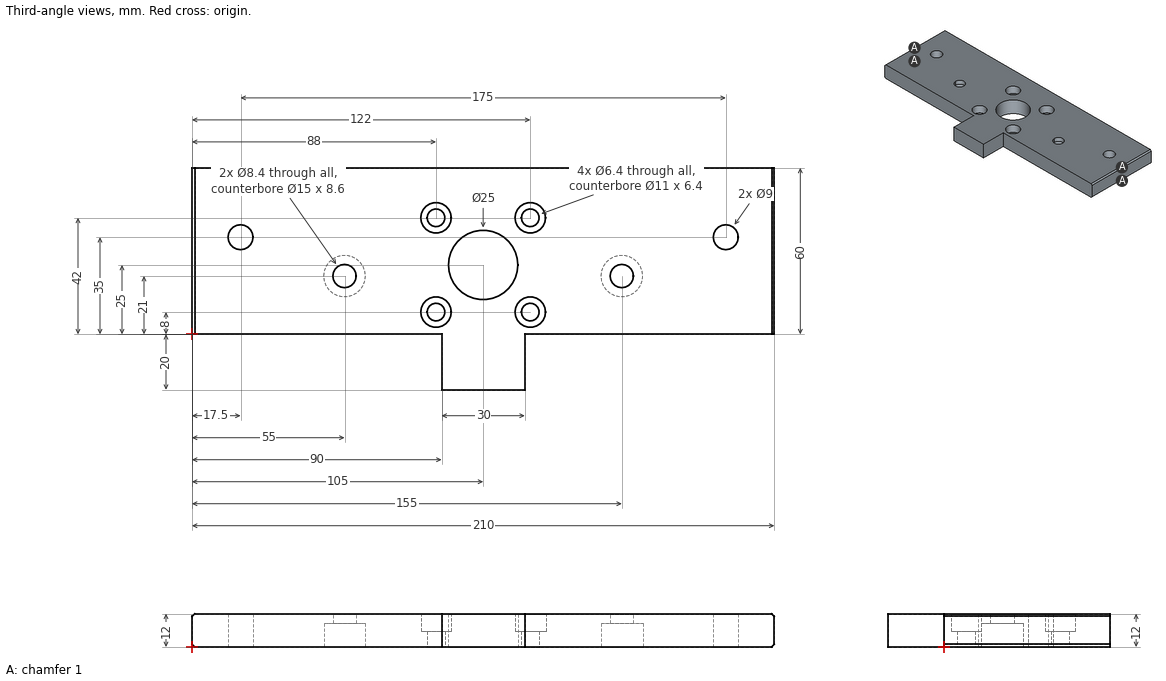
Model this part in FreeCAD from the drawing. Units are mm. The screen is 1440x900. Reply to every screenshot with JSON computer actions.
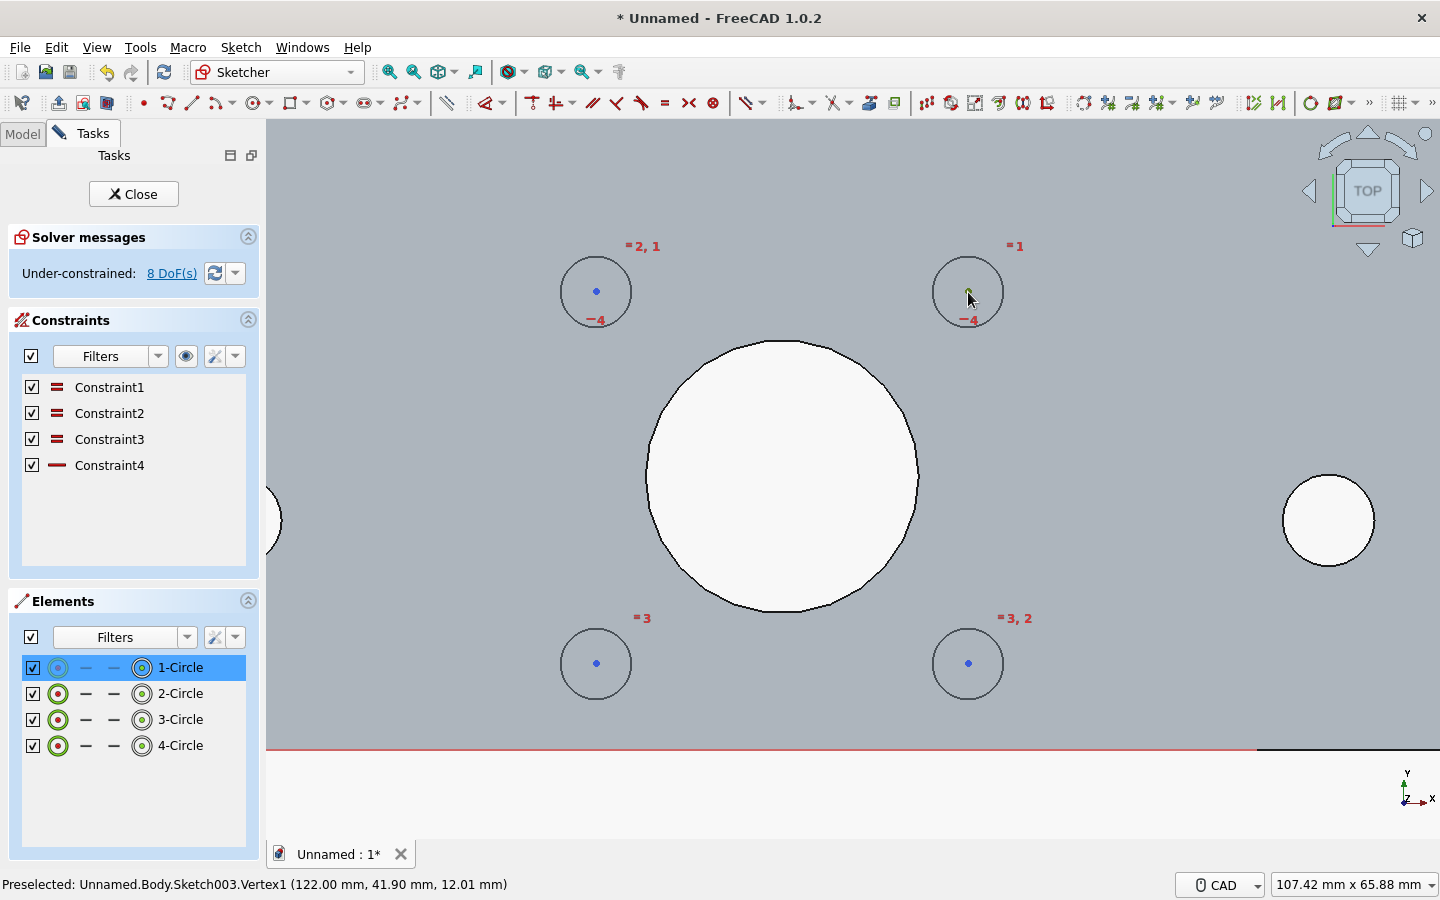
{"action": "left_click", "coordinate": [968, 664]}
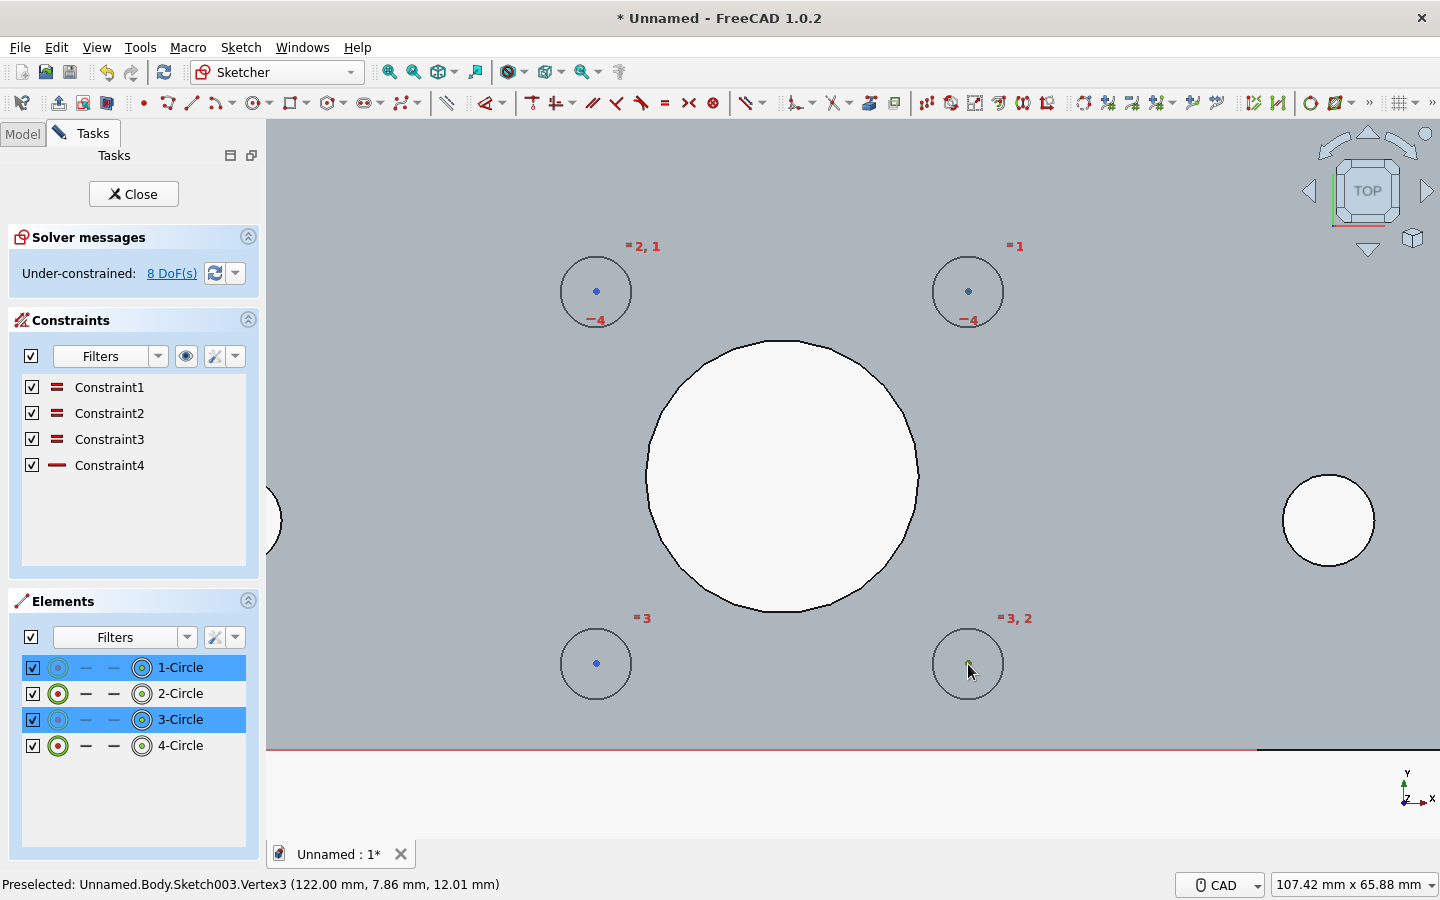
{"action": "key", "text": "v"}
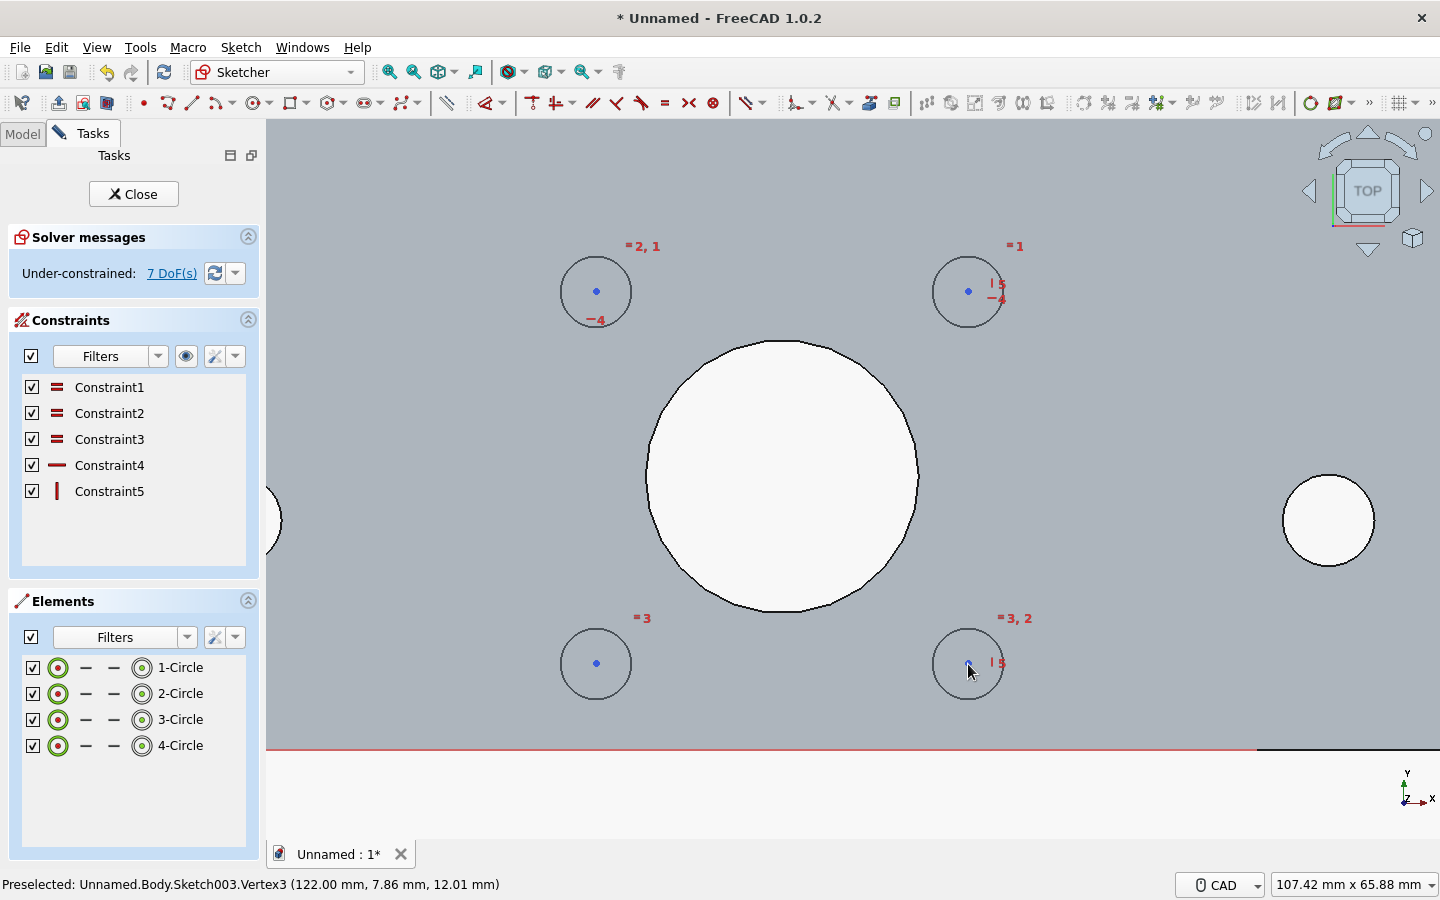
{"action": "left_click", "coordinate": [596, 292]}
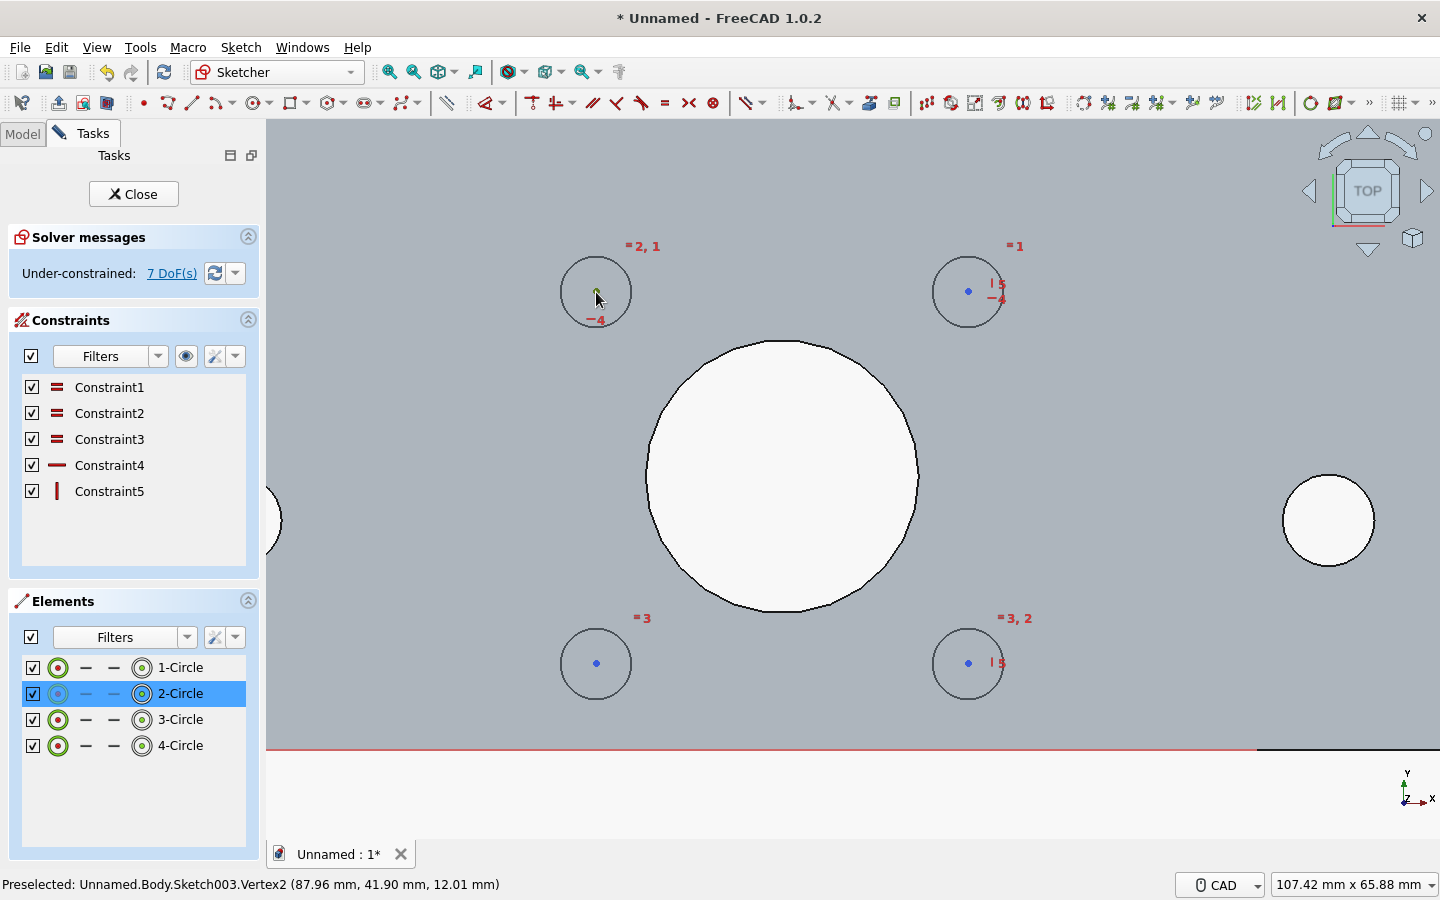
{"action": "left_click", "coordinate": [596, 664]}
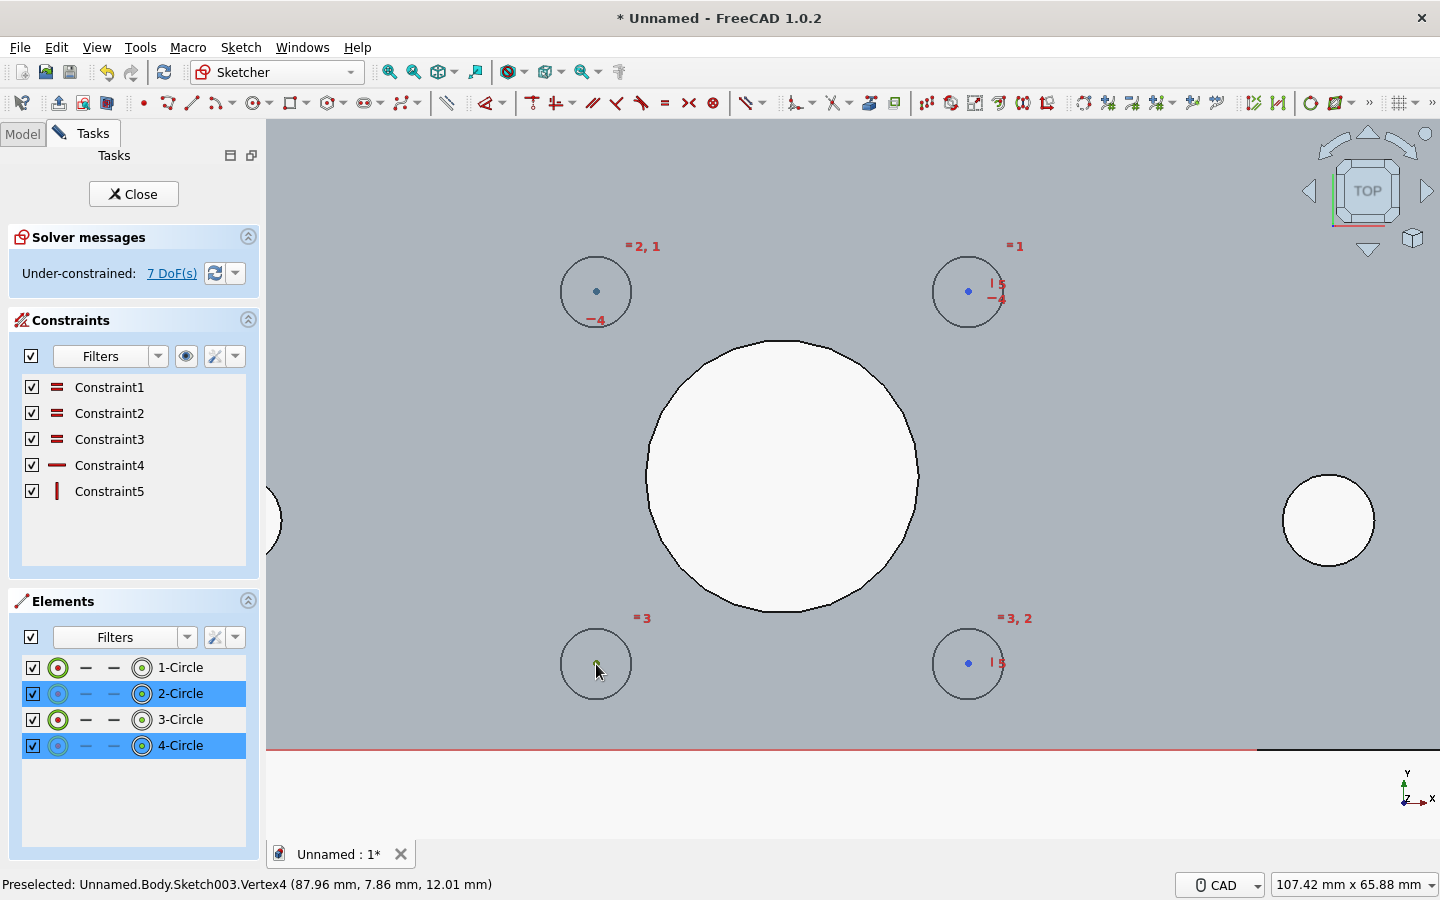
{"action": "key", "text": "v"}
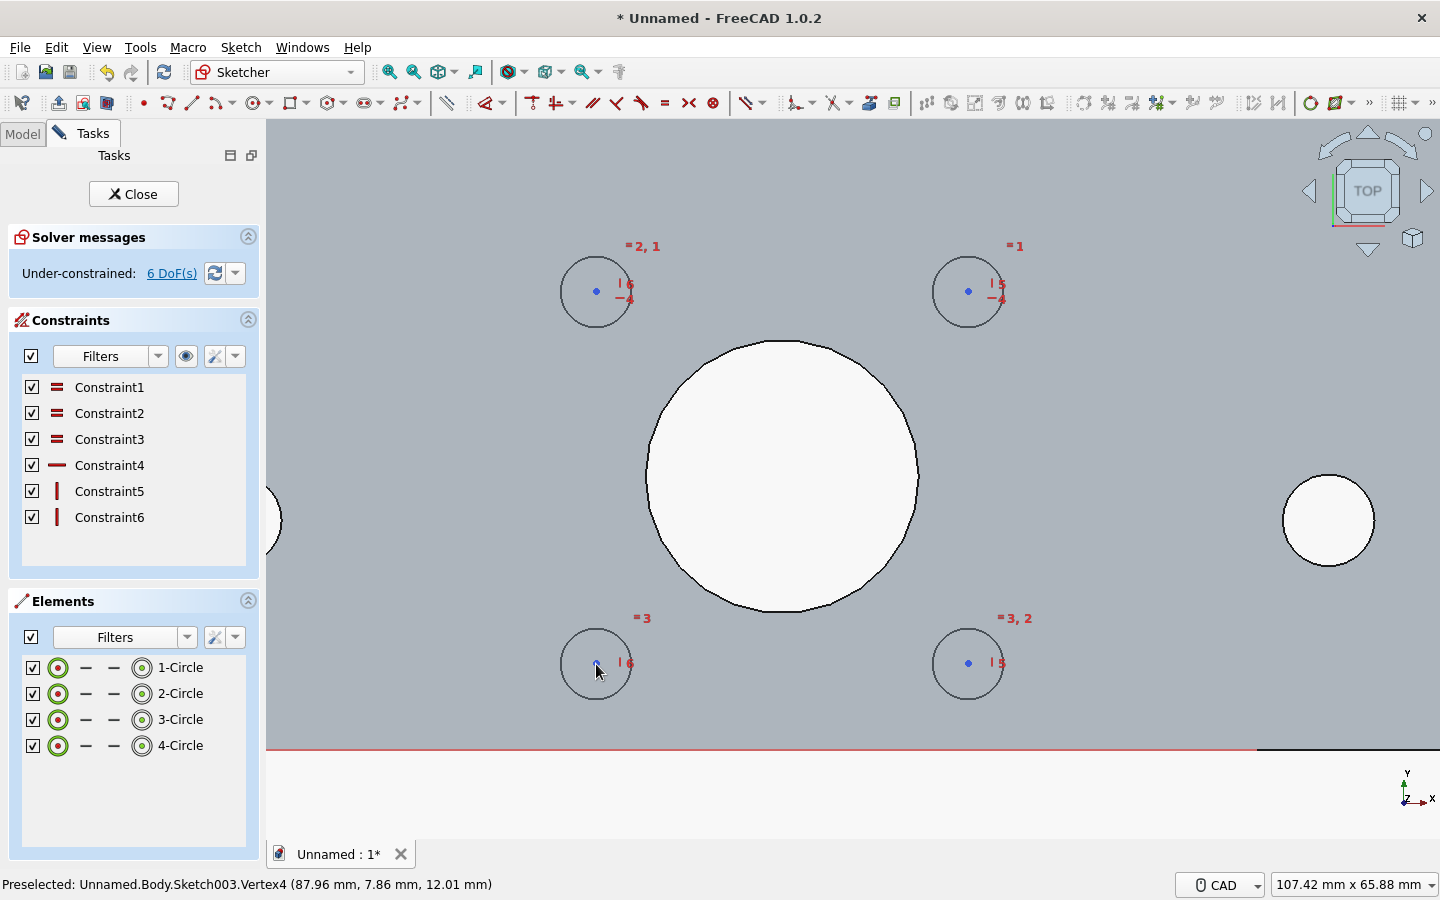
{"action": "left_click", "coordinate": [968, 664]}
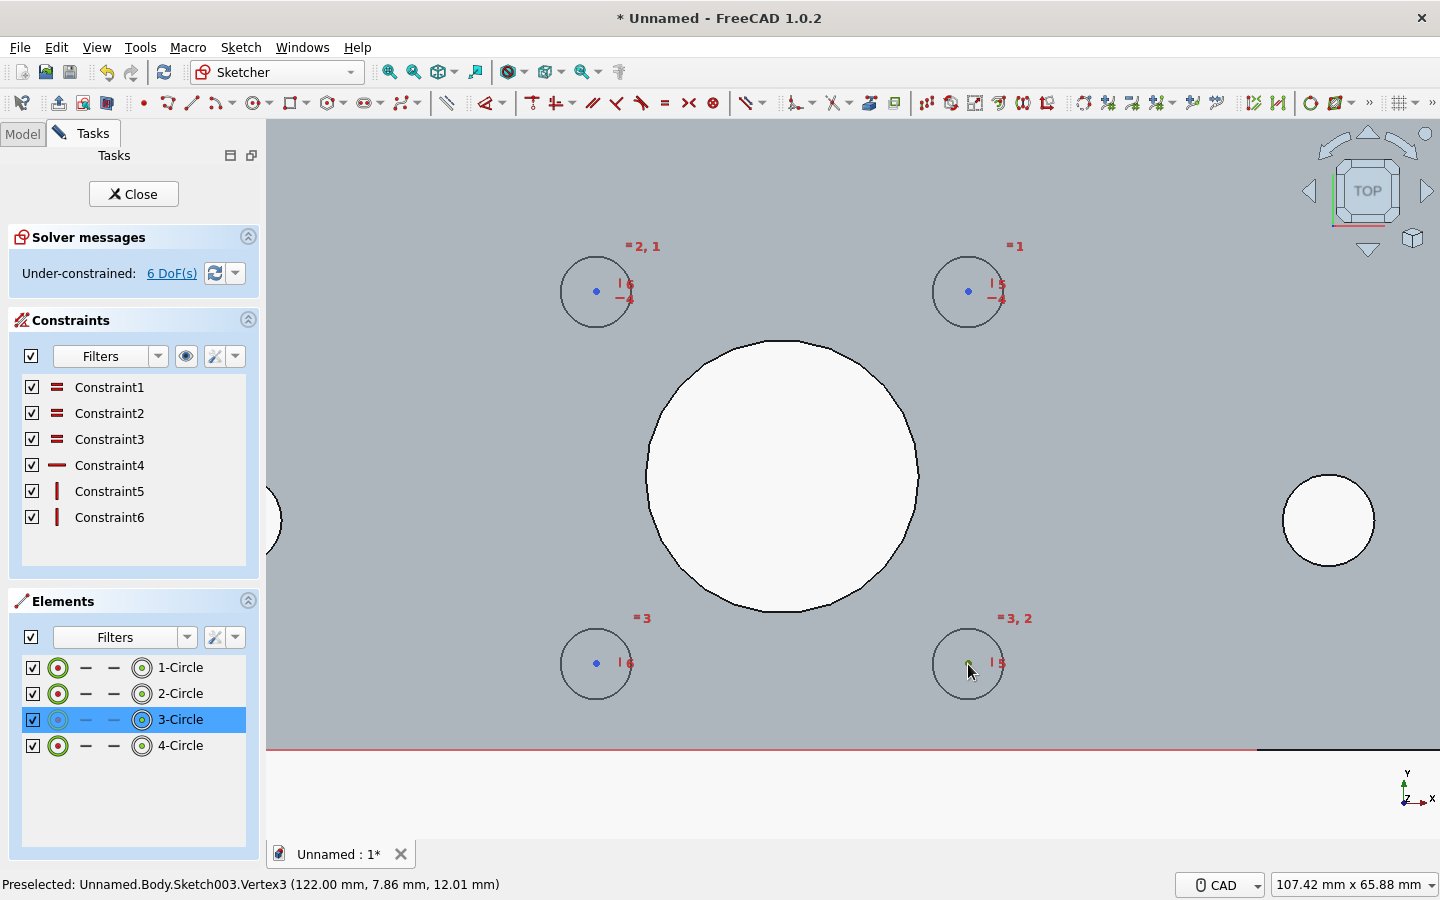
{"action": "left_click", "coordinate": [596, 664]}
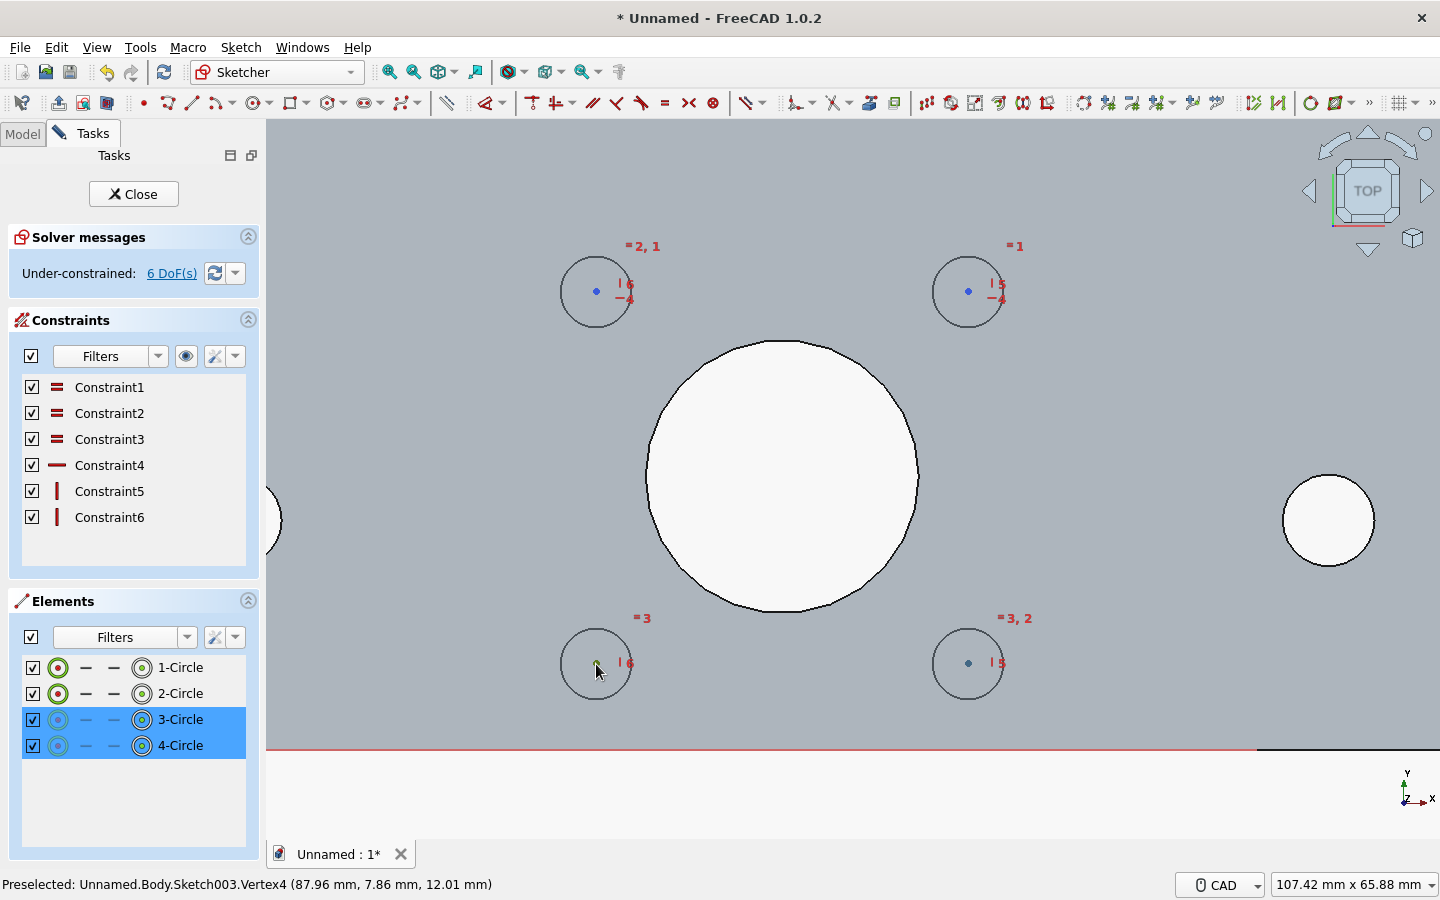
{"action": "key", "text": "h"}